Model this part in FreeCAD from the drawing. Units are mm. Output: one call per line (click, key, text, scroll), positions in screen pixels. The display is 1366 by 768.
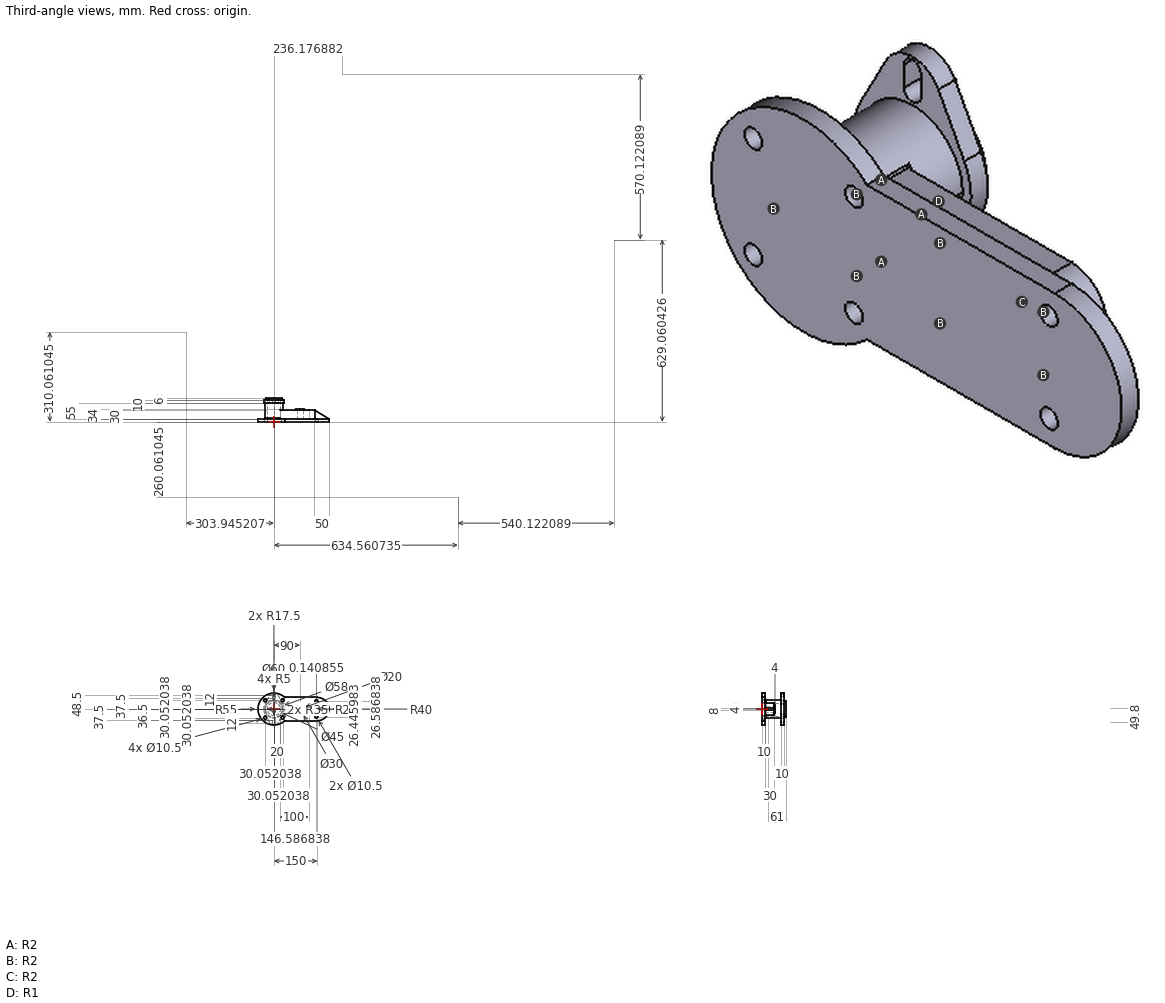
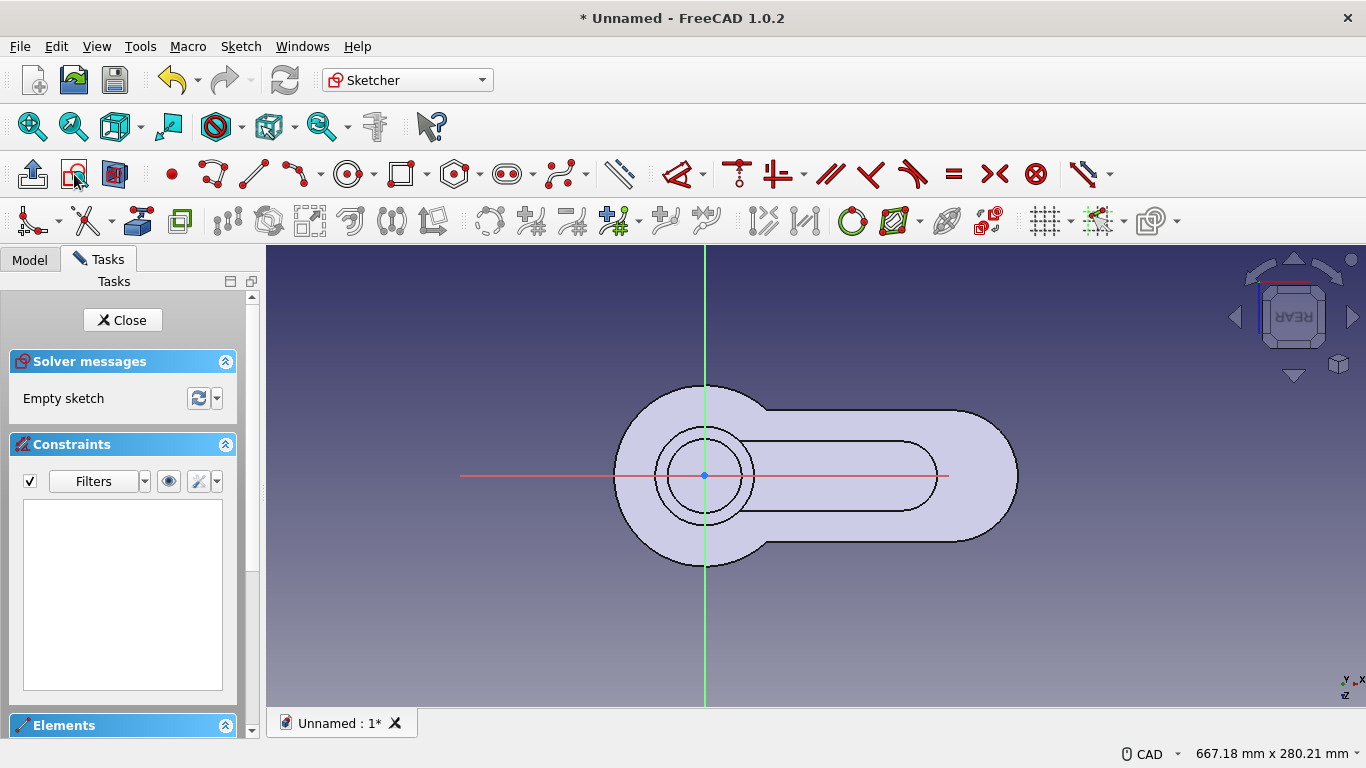
scroll(874, 476, up, 9)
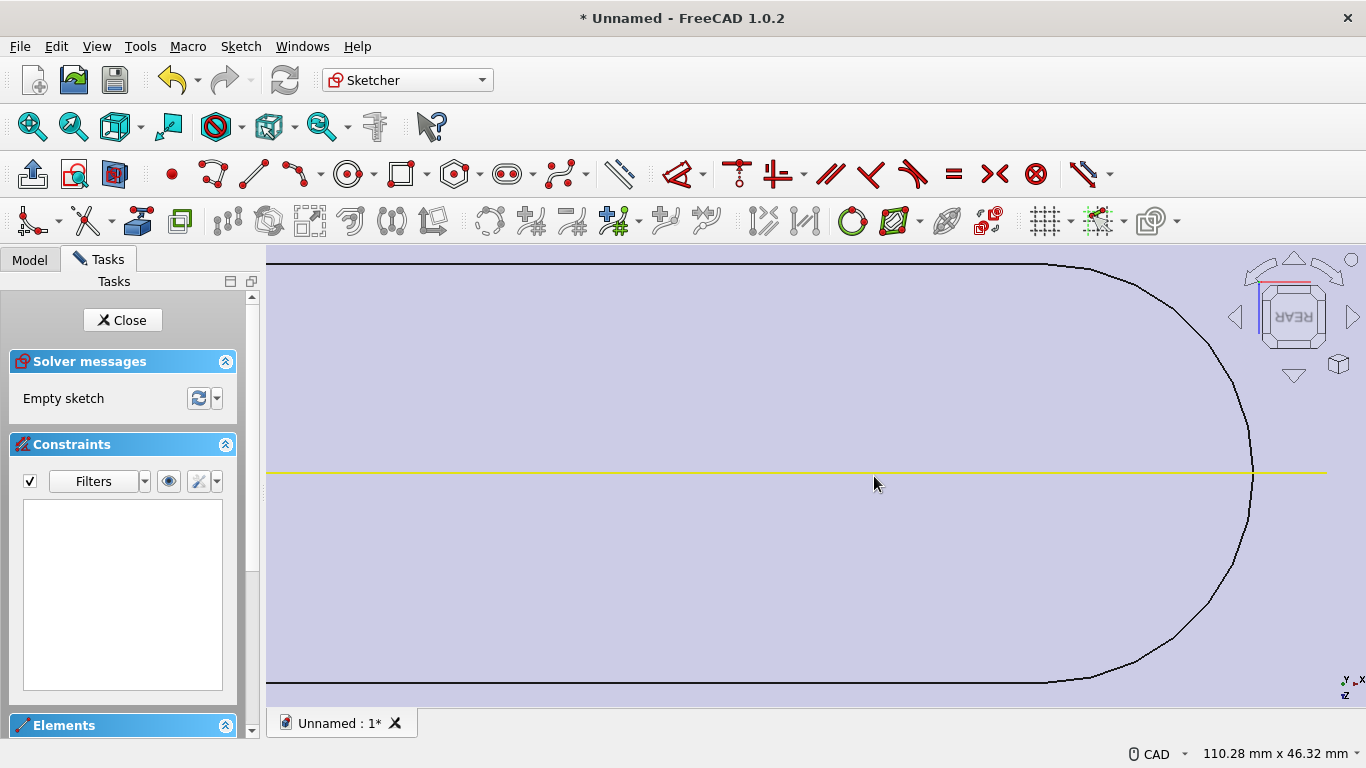
key(g)
key(c)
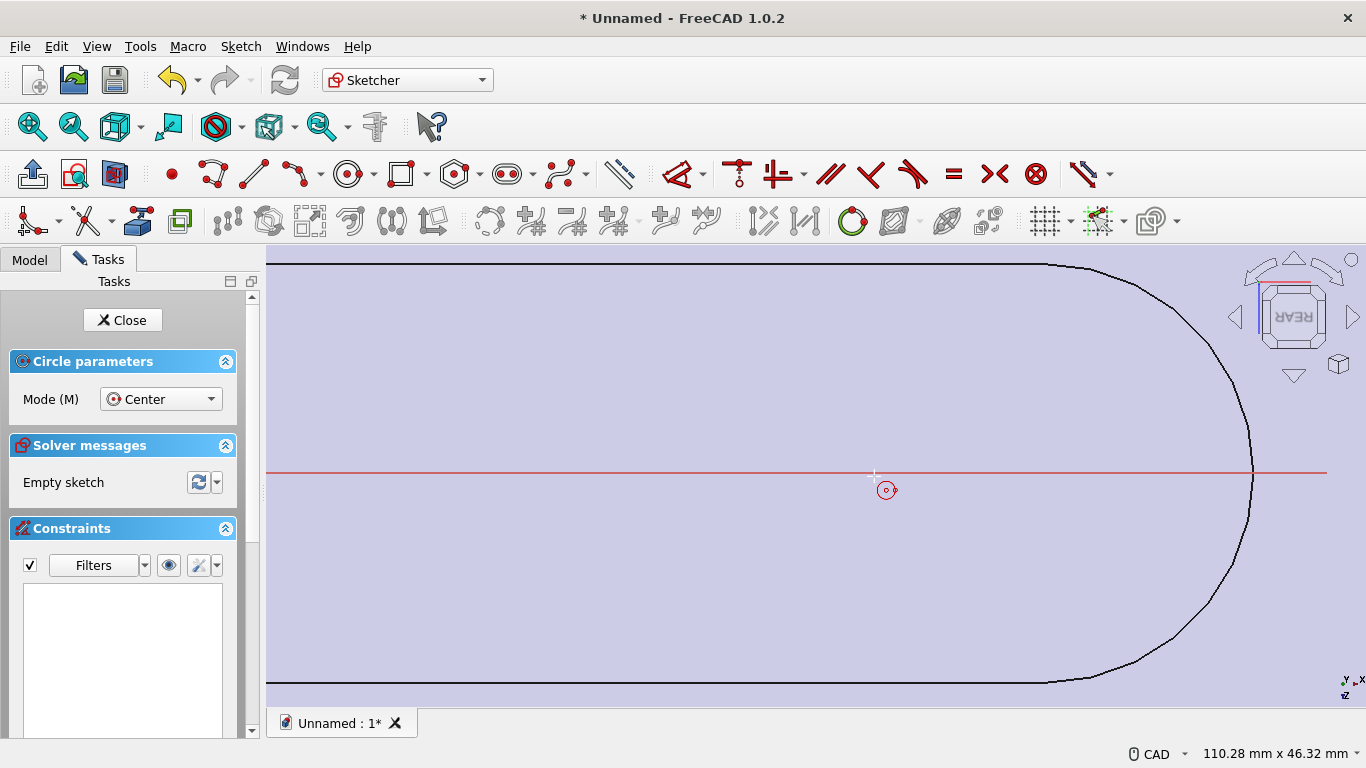
click(745, 473)
click(851, 368)
key(Escape)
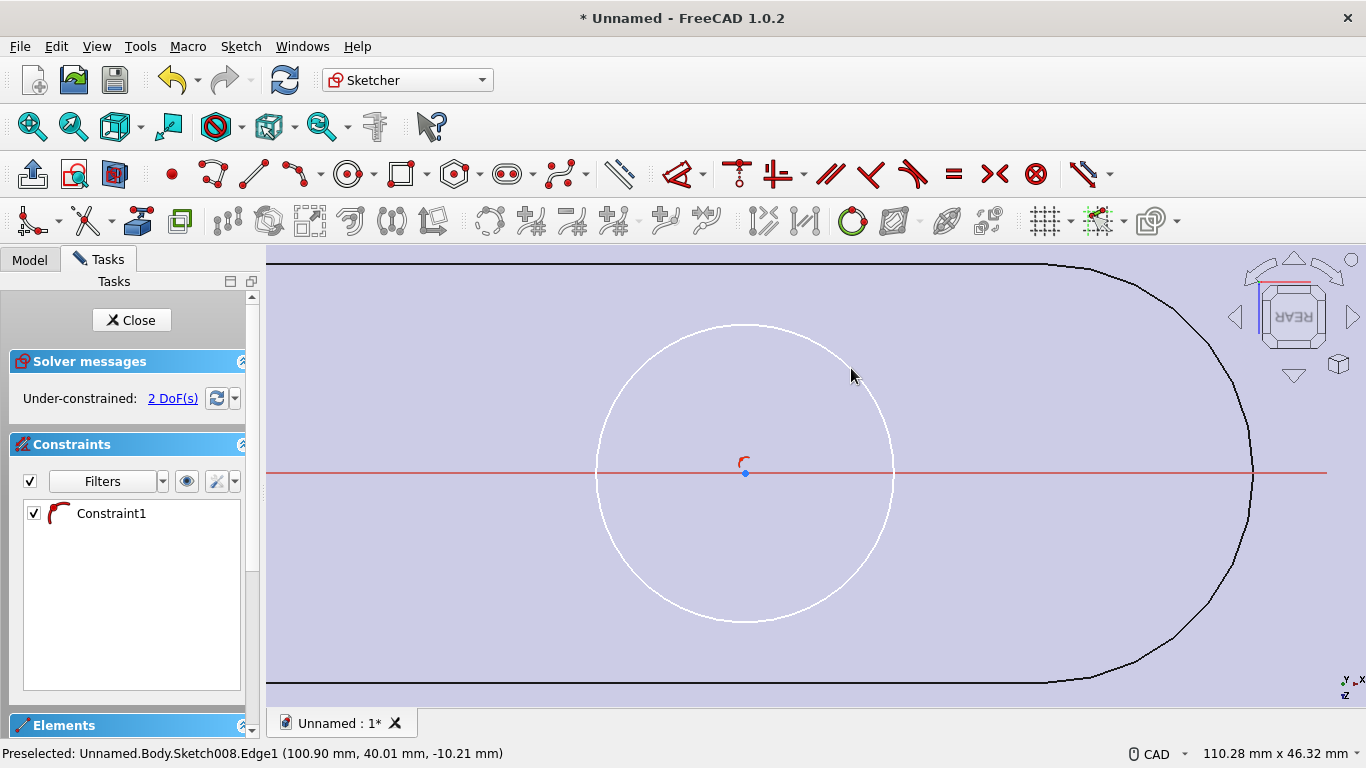
key(d)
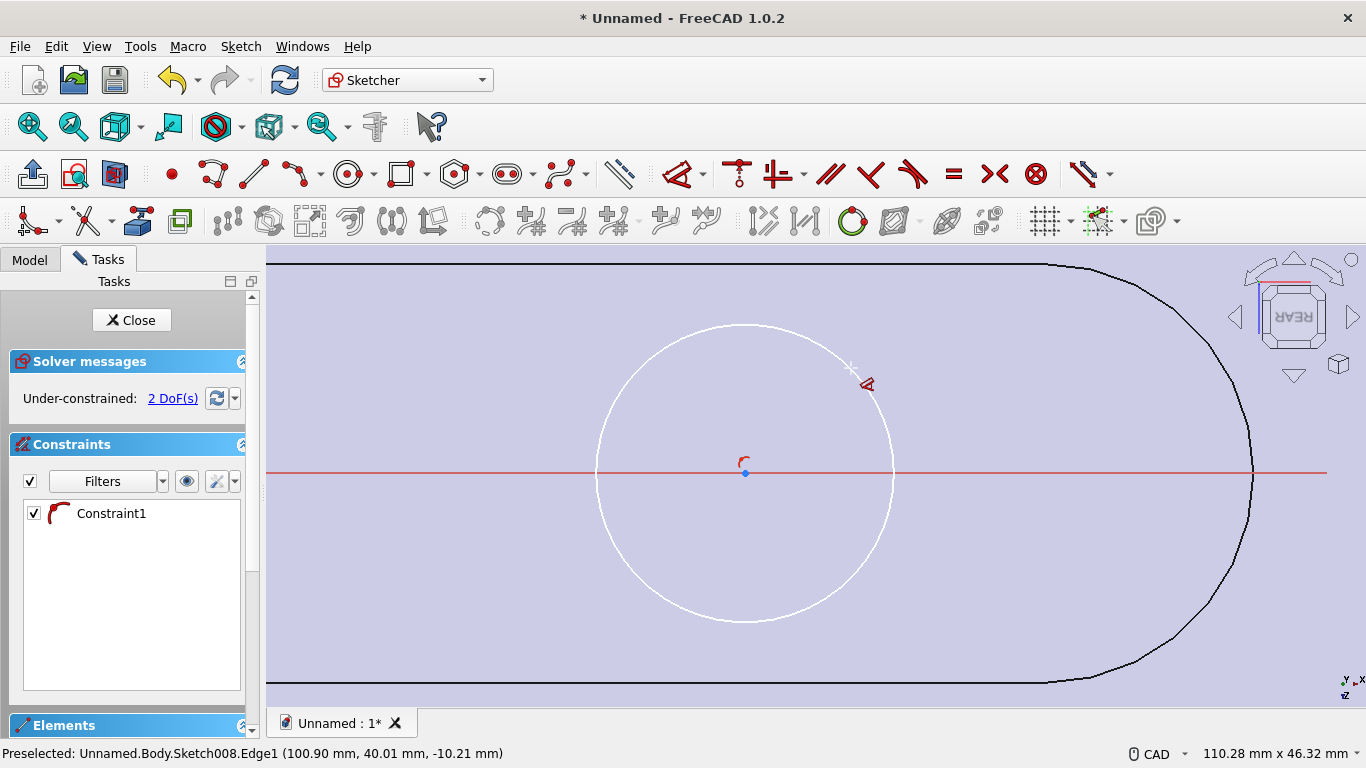
click(850, 368)
click(873, 345)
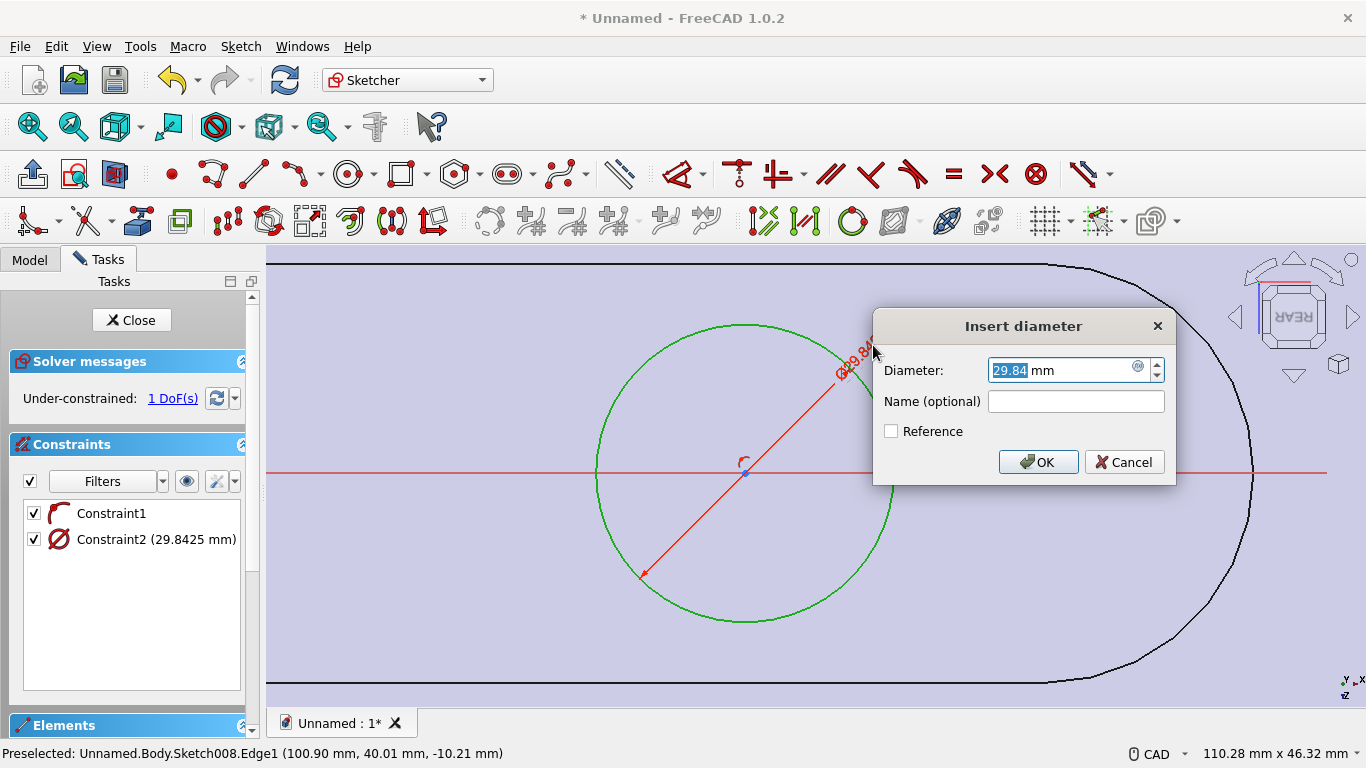
text(30)
key(Return)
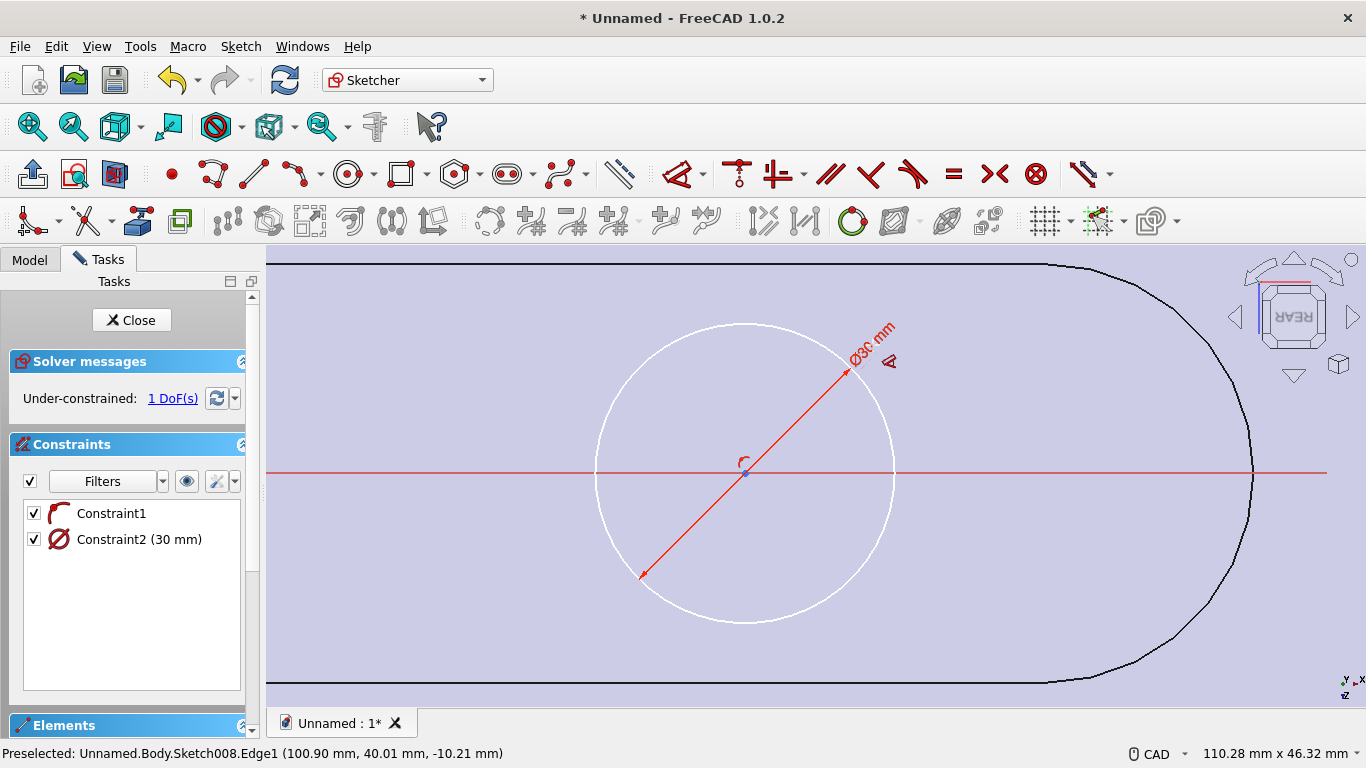
click(745, 473)
click(519, 507)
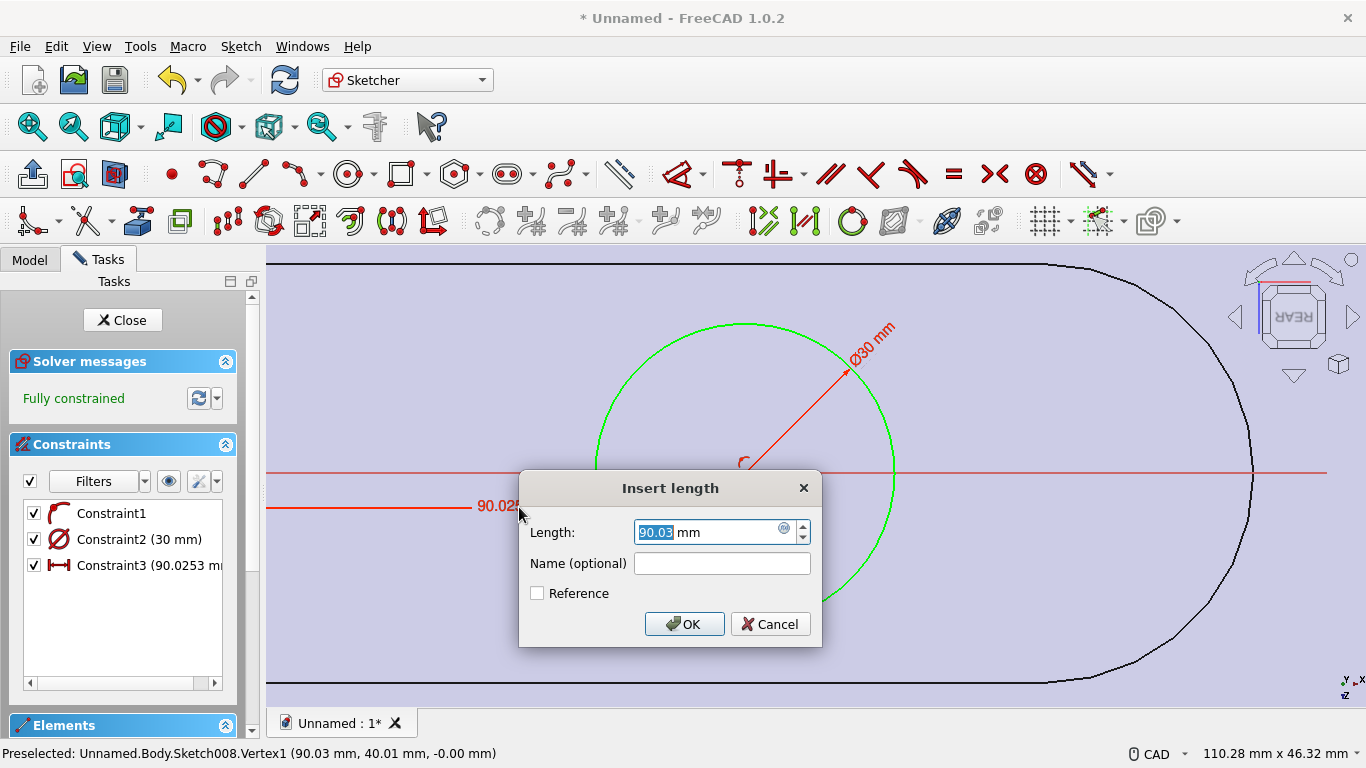
text(90)
key(Return)
key(Escape)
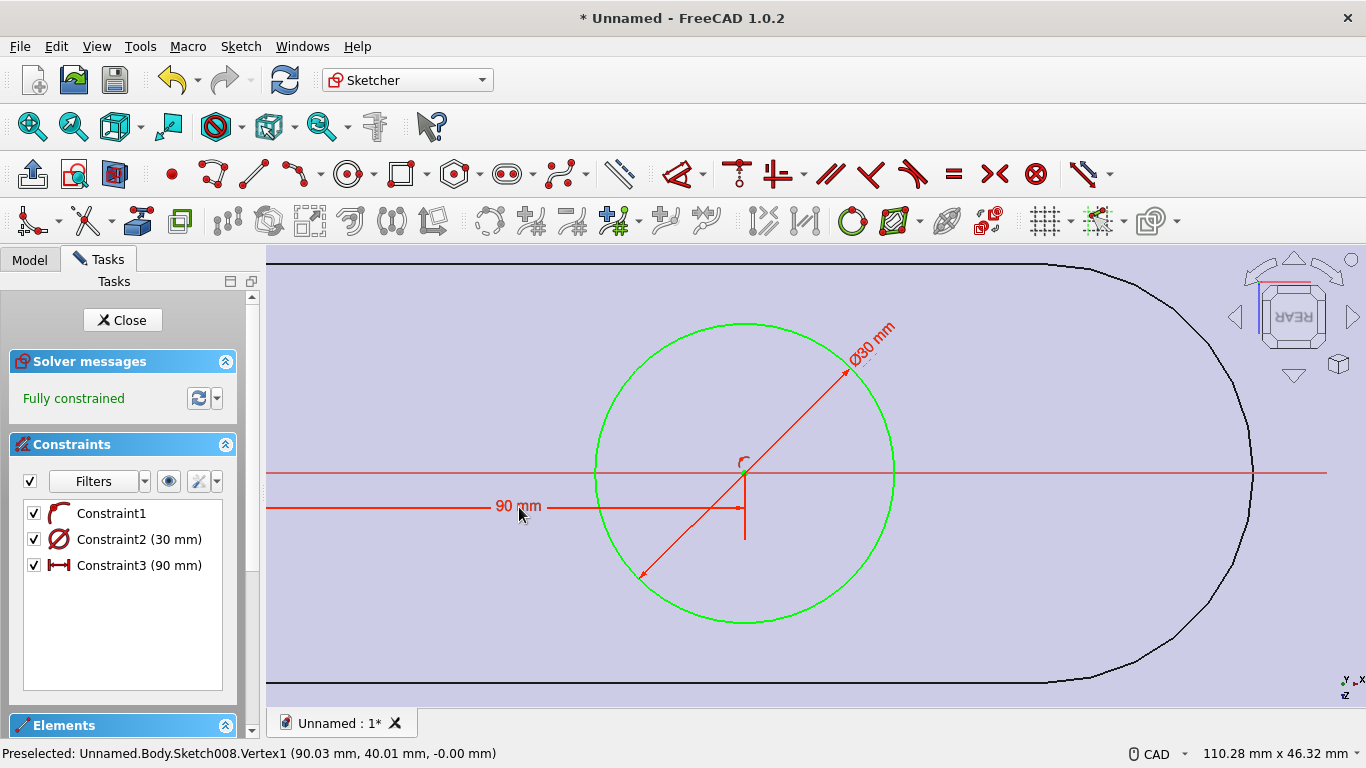
click(123, 320)